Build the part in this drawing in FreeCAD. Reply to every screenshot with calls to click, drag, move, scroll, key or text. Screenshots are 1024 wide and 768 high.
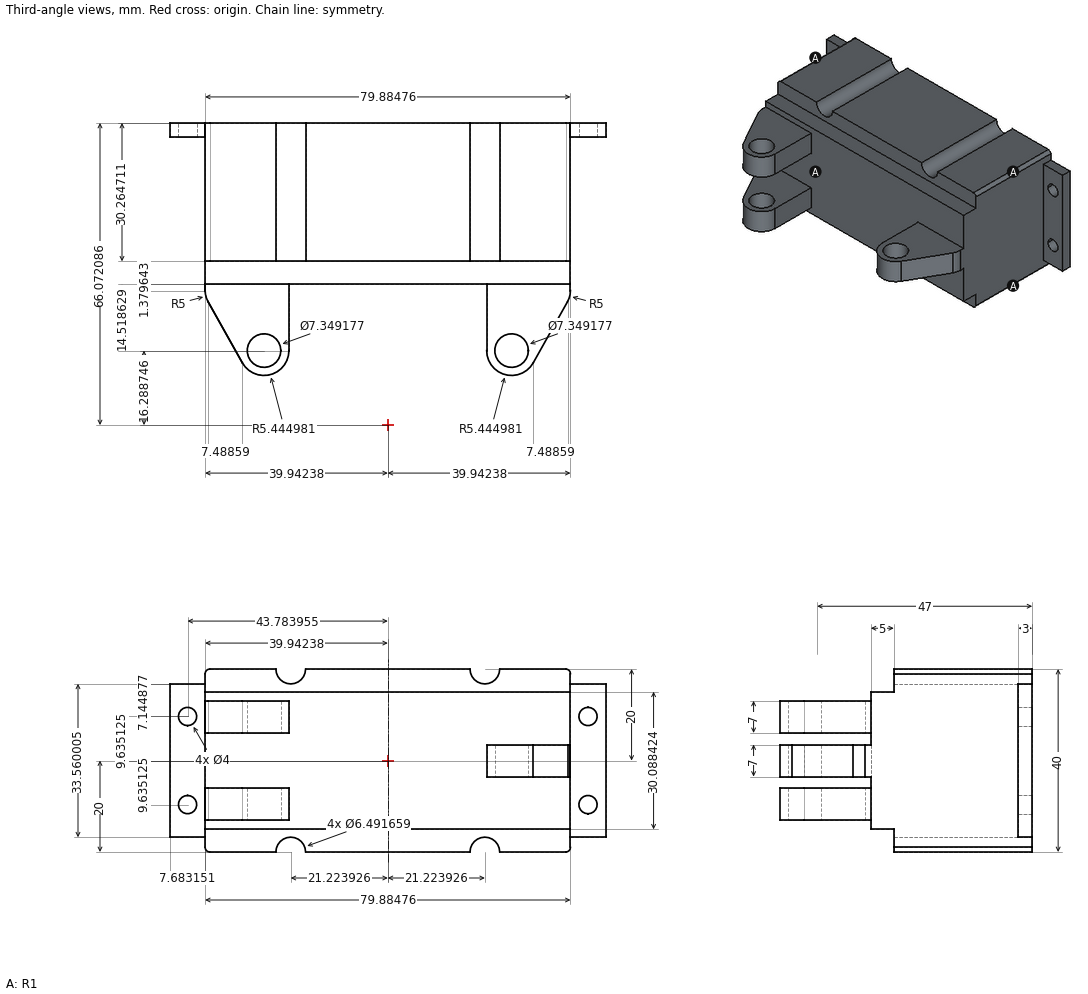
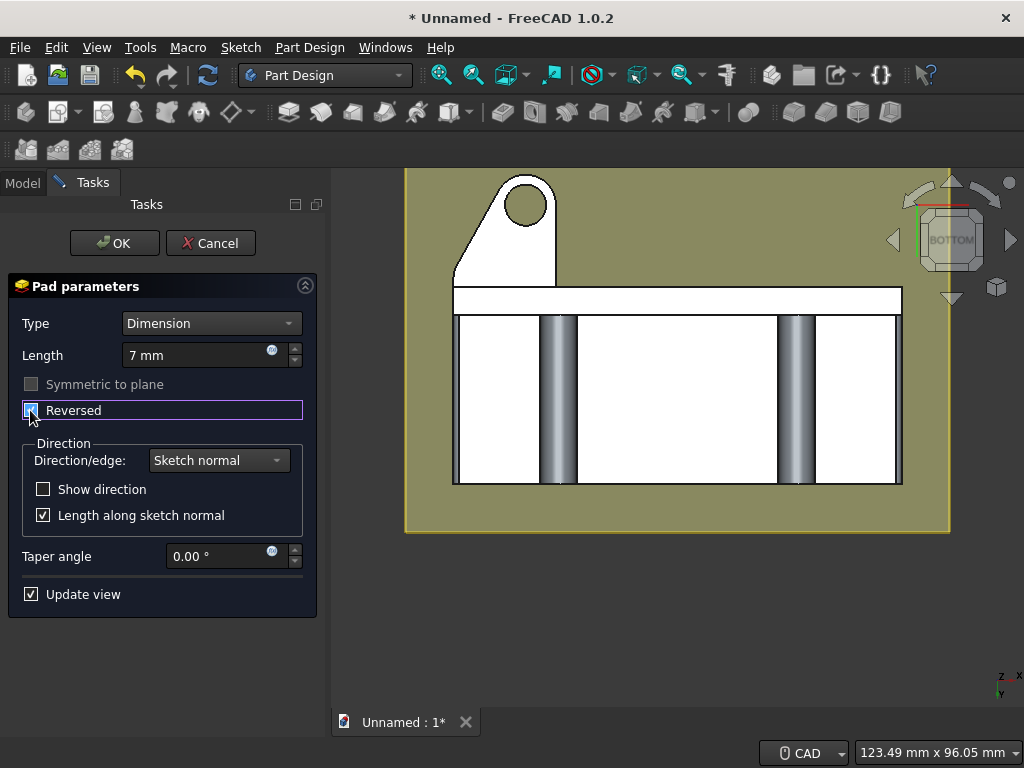
click(115, 243)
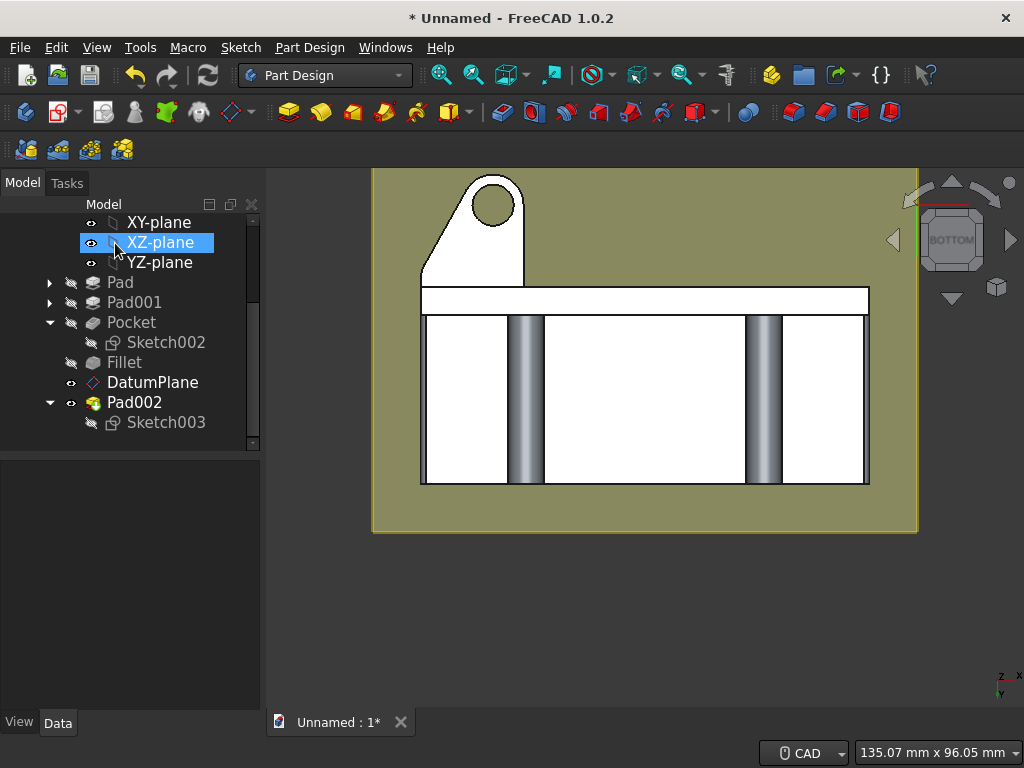
click(116, 383)
key(space)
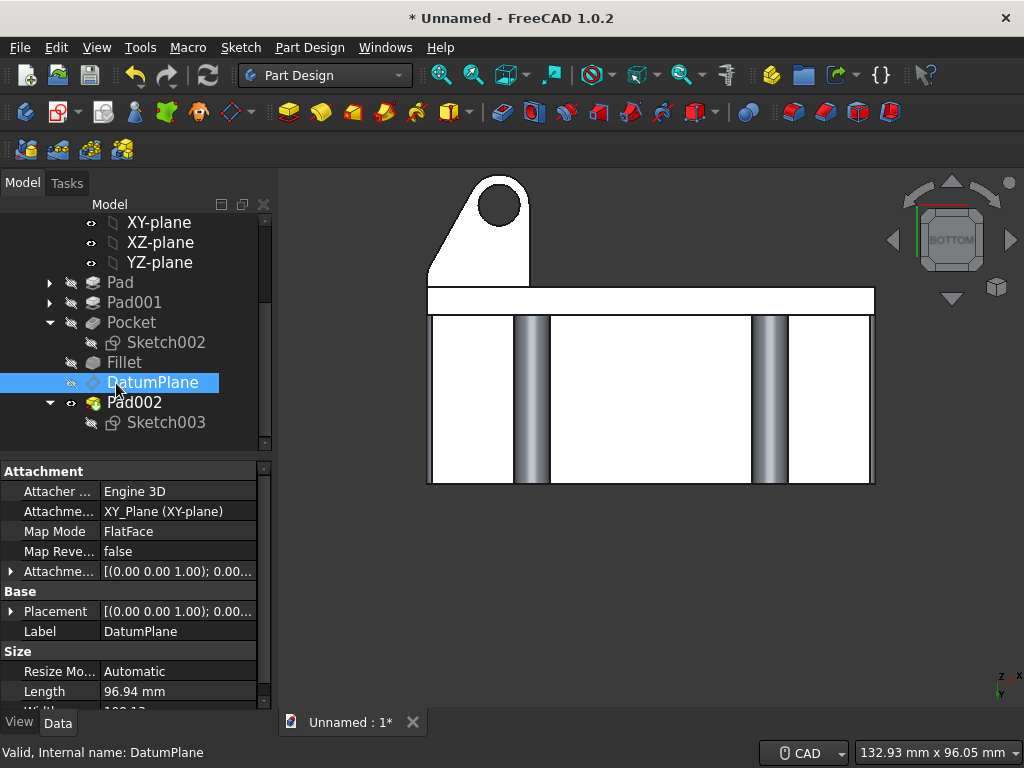
click(116, 403)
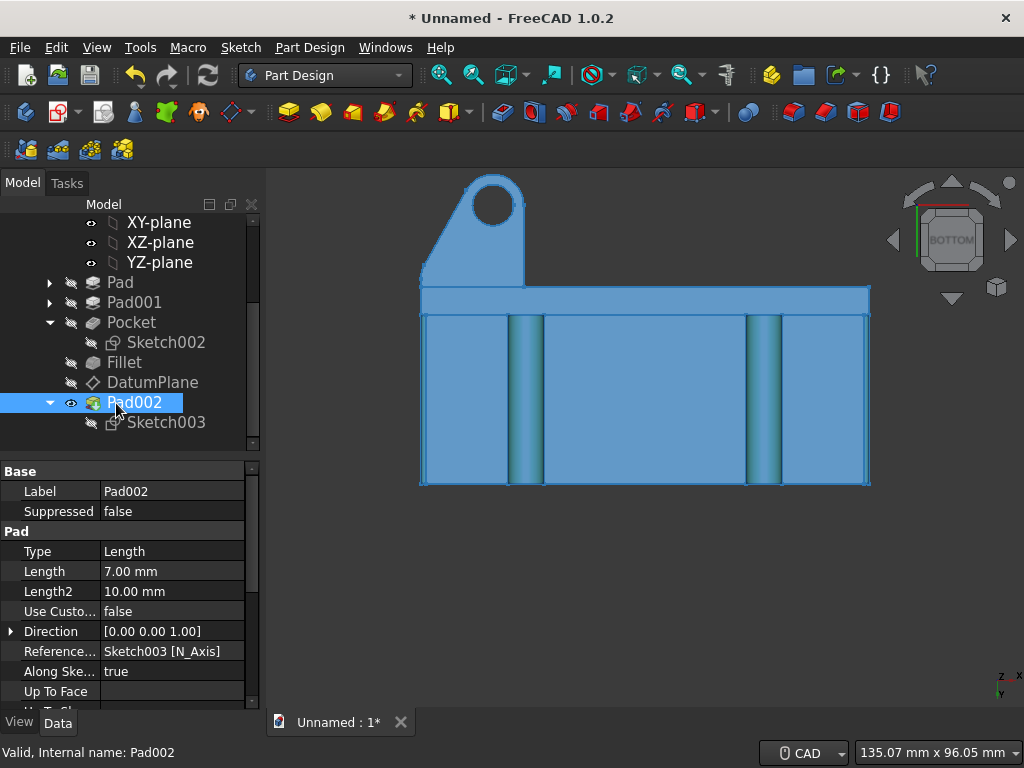
click(26, 150)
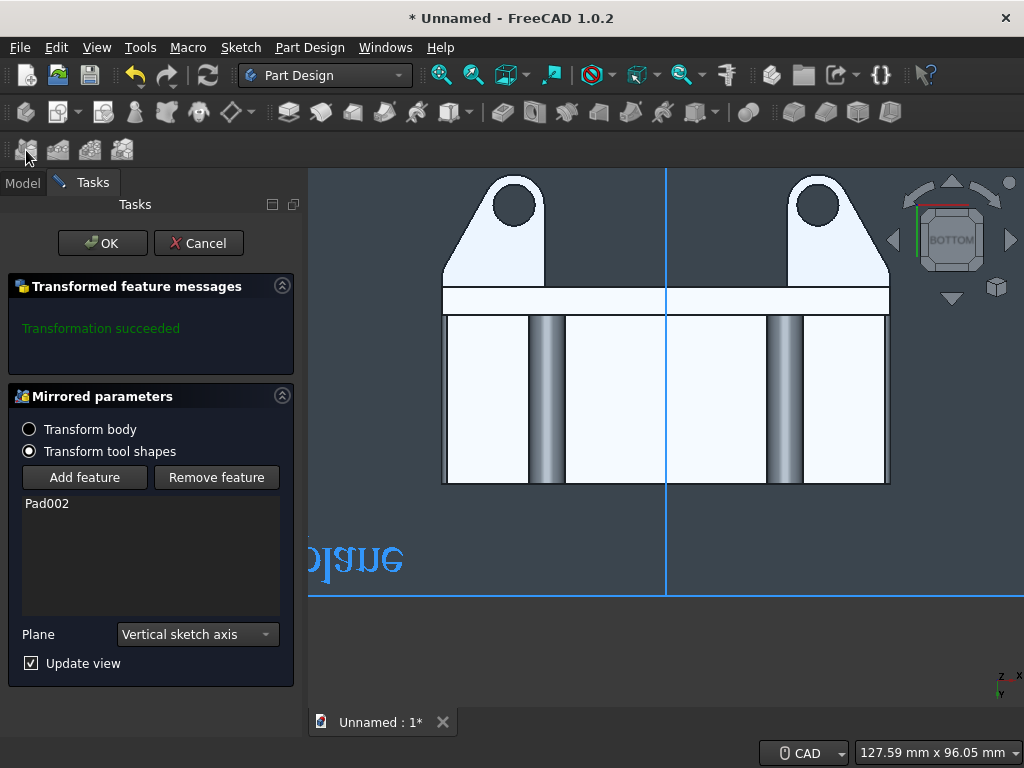
click(198, 634)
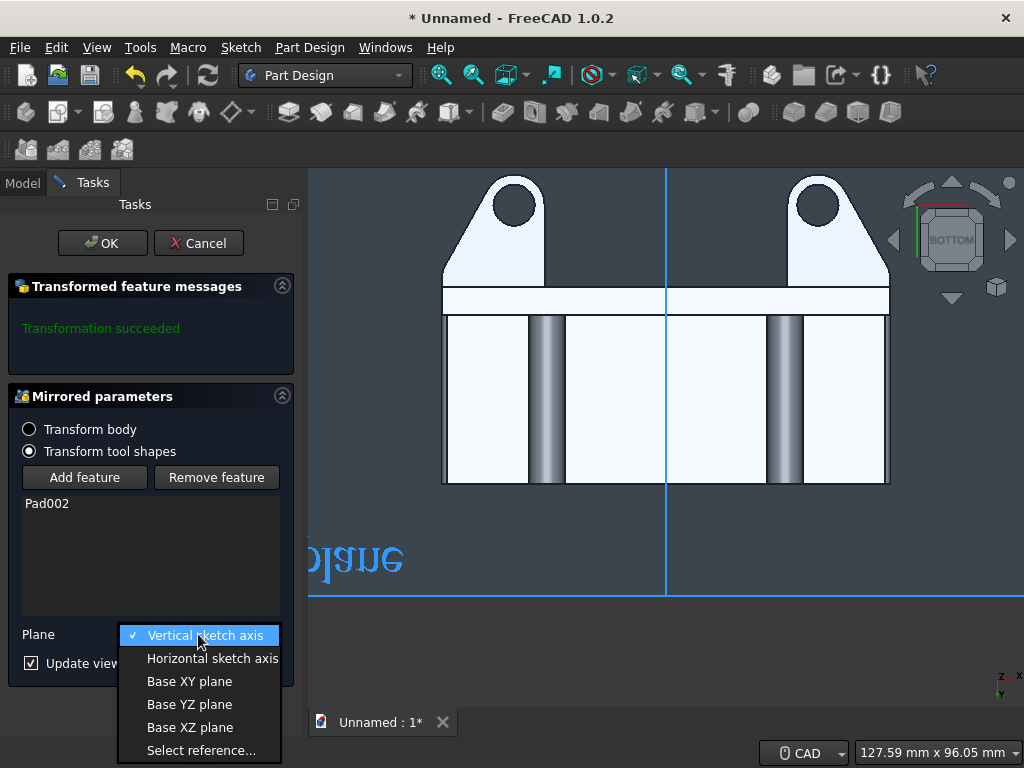
click(198, 682)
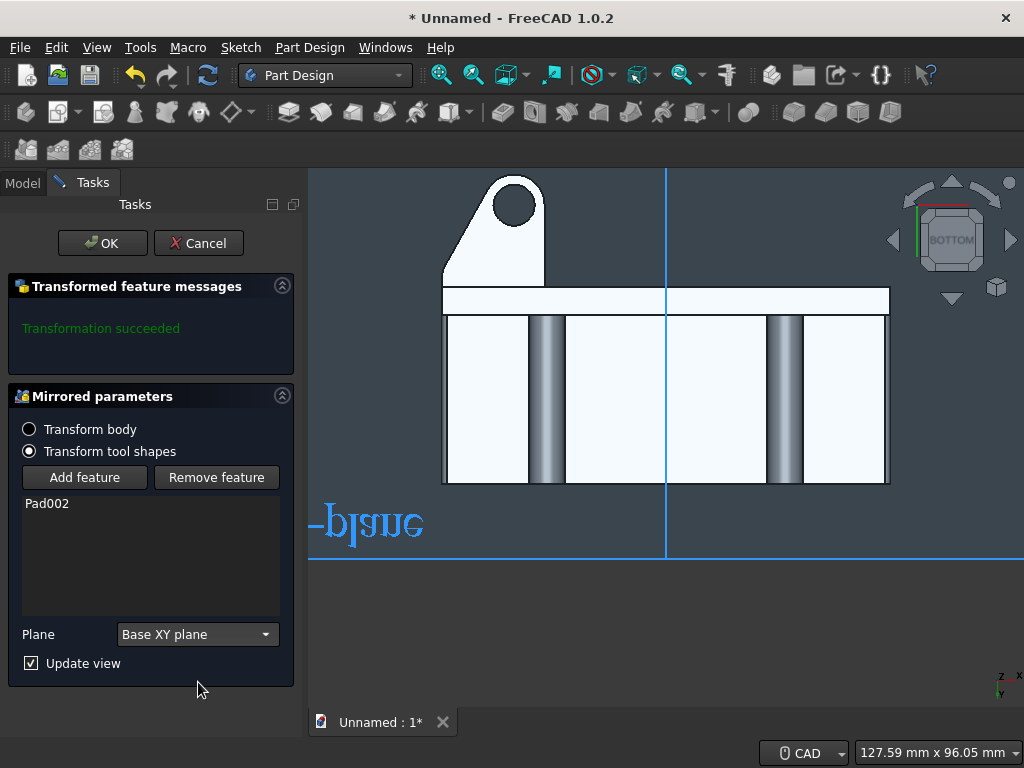
click(103, 243)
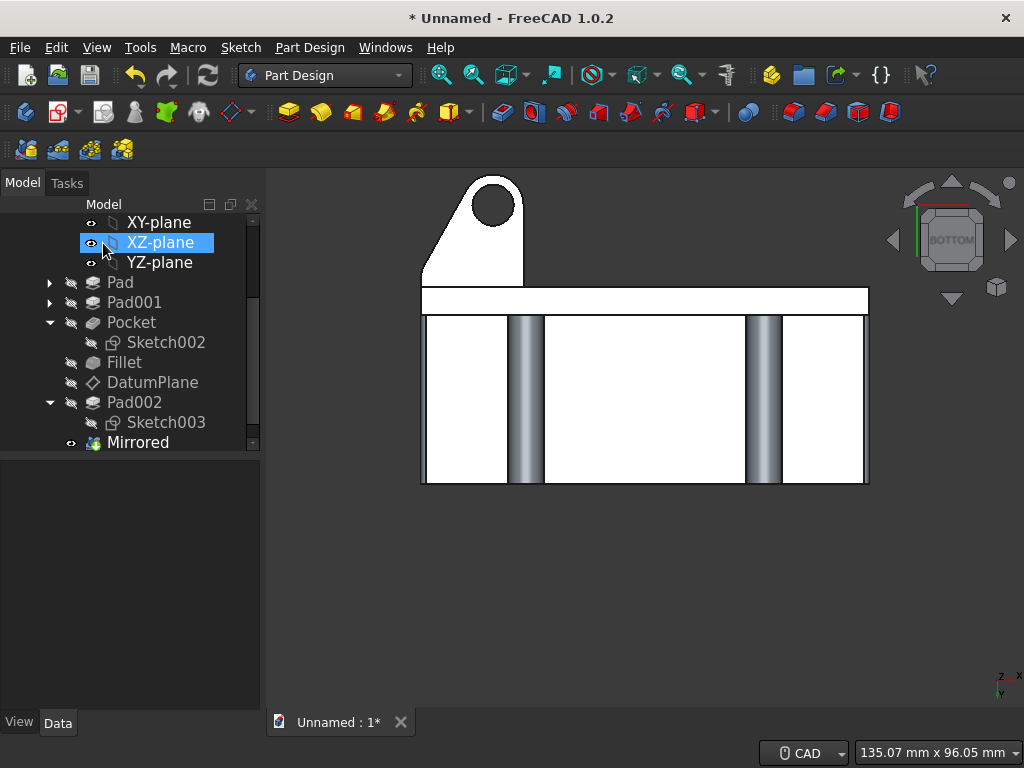
click(58, 112)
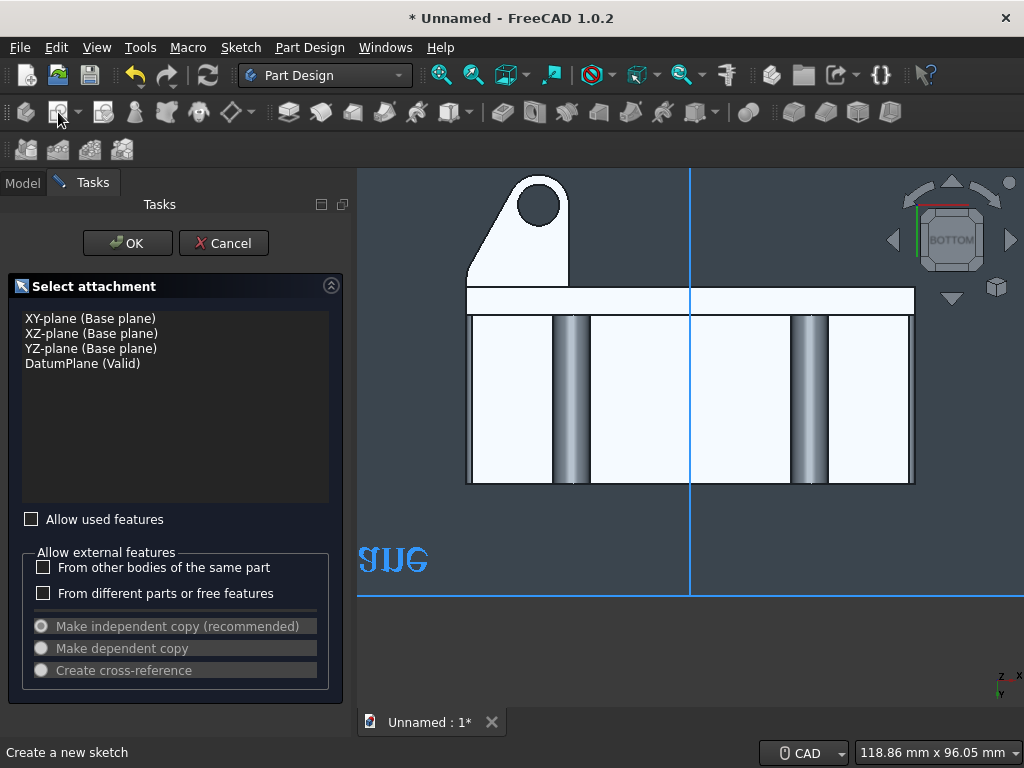
click(82, 318)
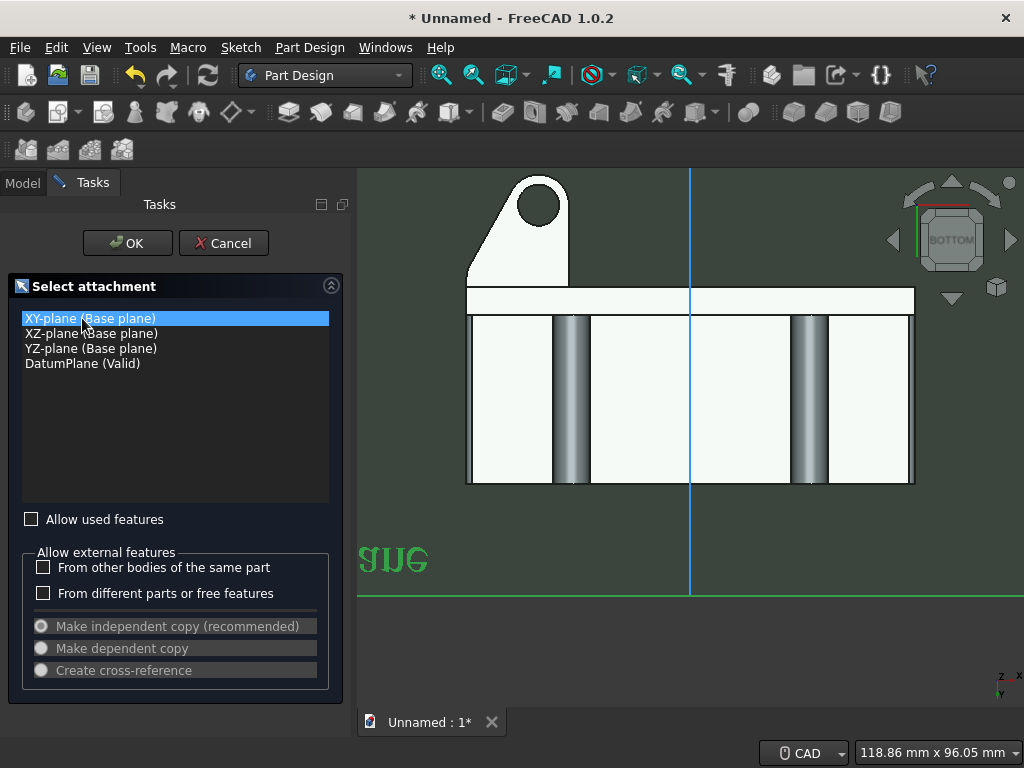
click(128, 243)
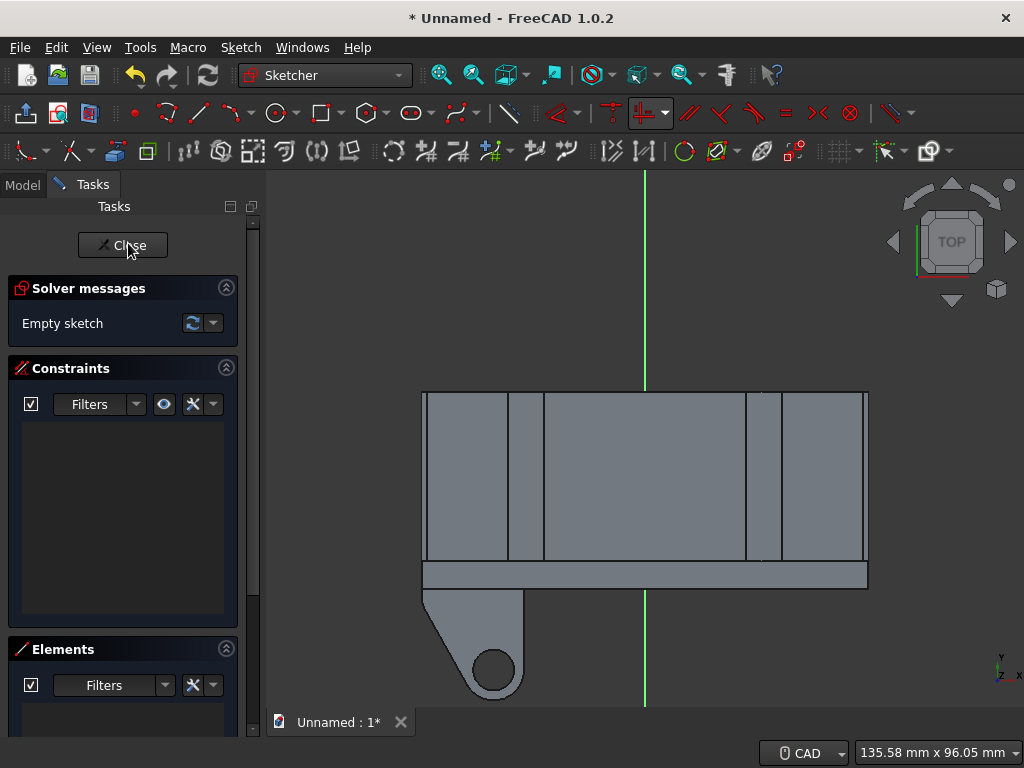
click(90, 114)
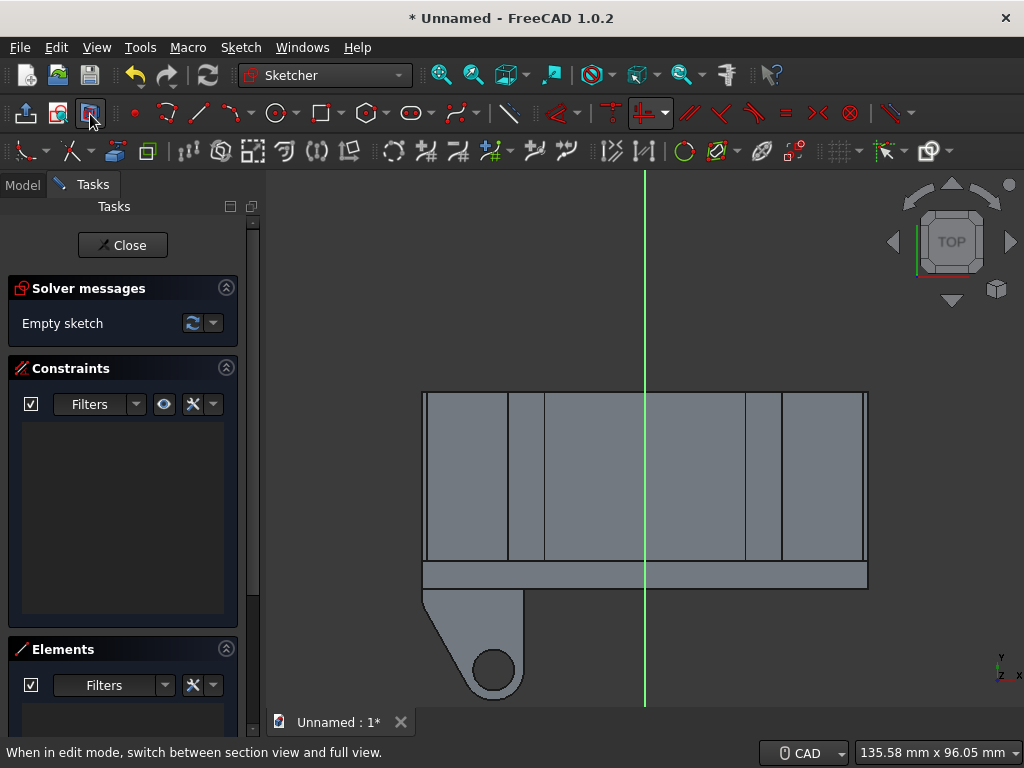
scroll(576, 438, down, 5)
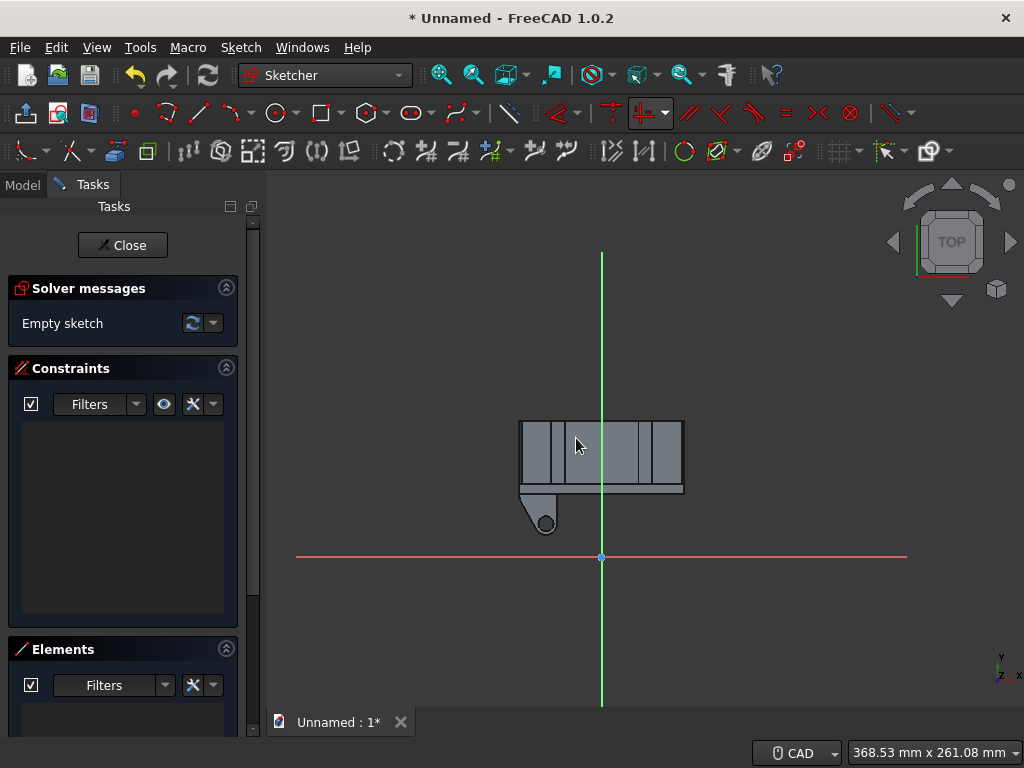
scroll(659, 548, up, 8)